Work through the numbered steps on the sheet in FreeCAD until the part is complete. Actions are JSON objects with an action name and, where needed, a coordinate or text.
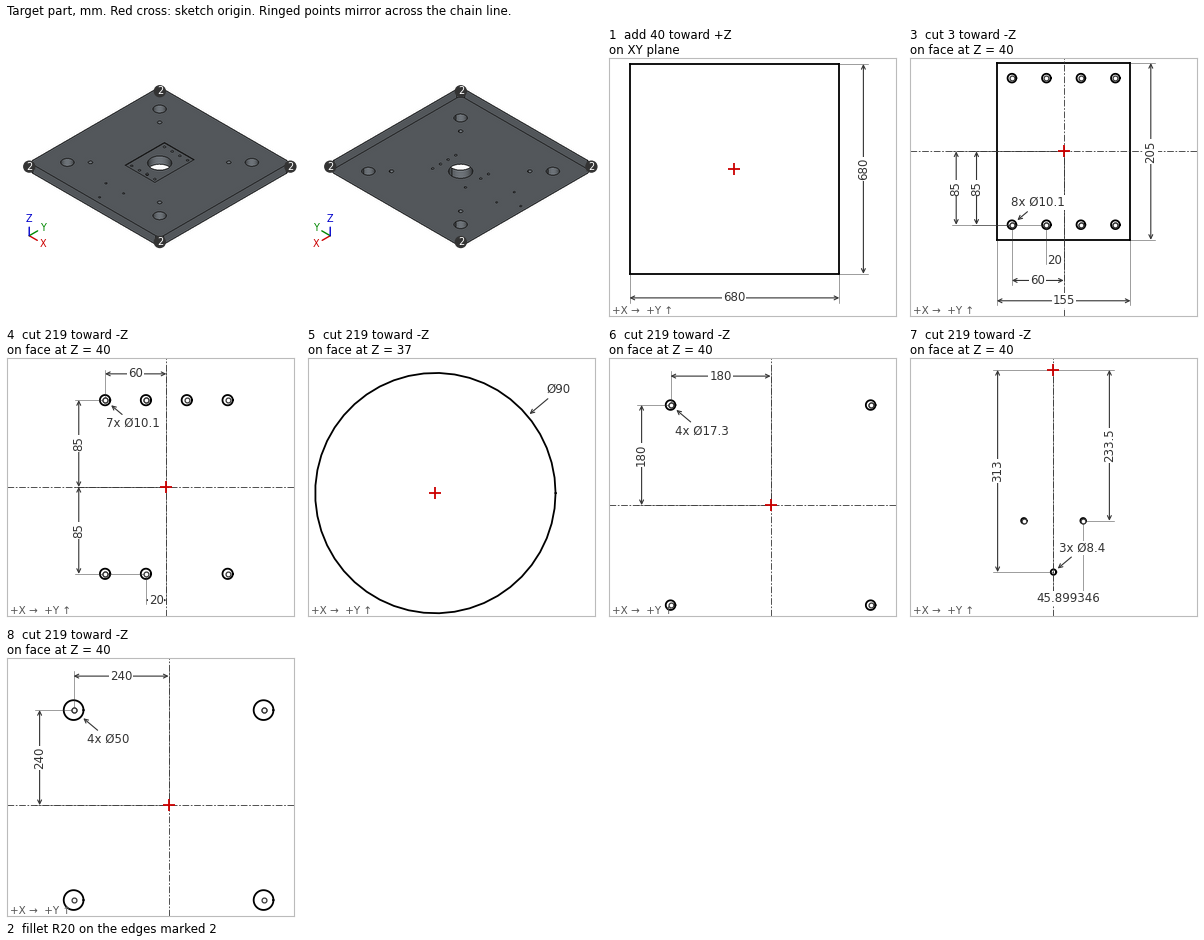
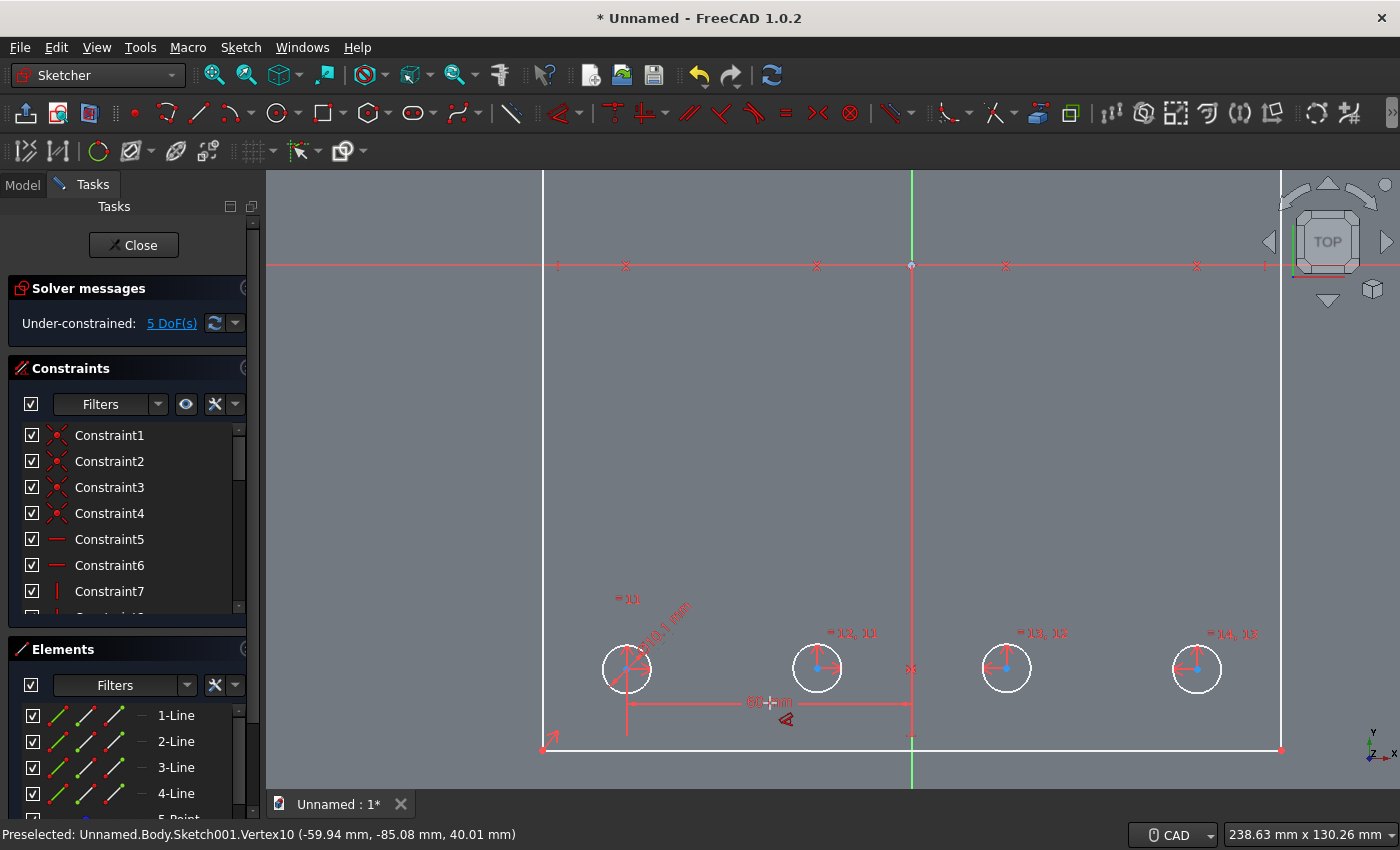
{"action": "left_click", "coordinate": [627, 669]}
{"action": "left_click", "coordinate": [593, 467]}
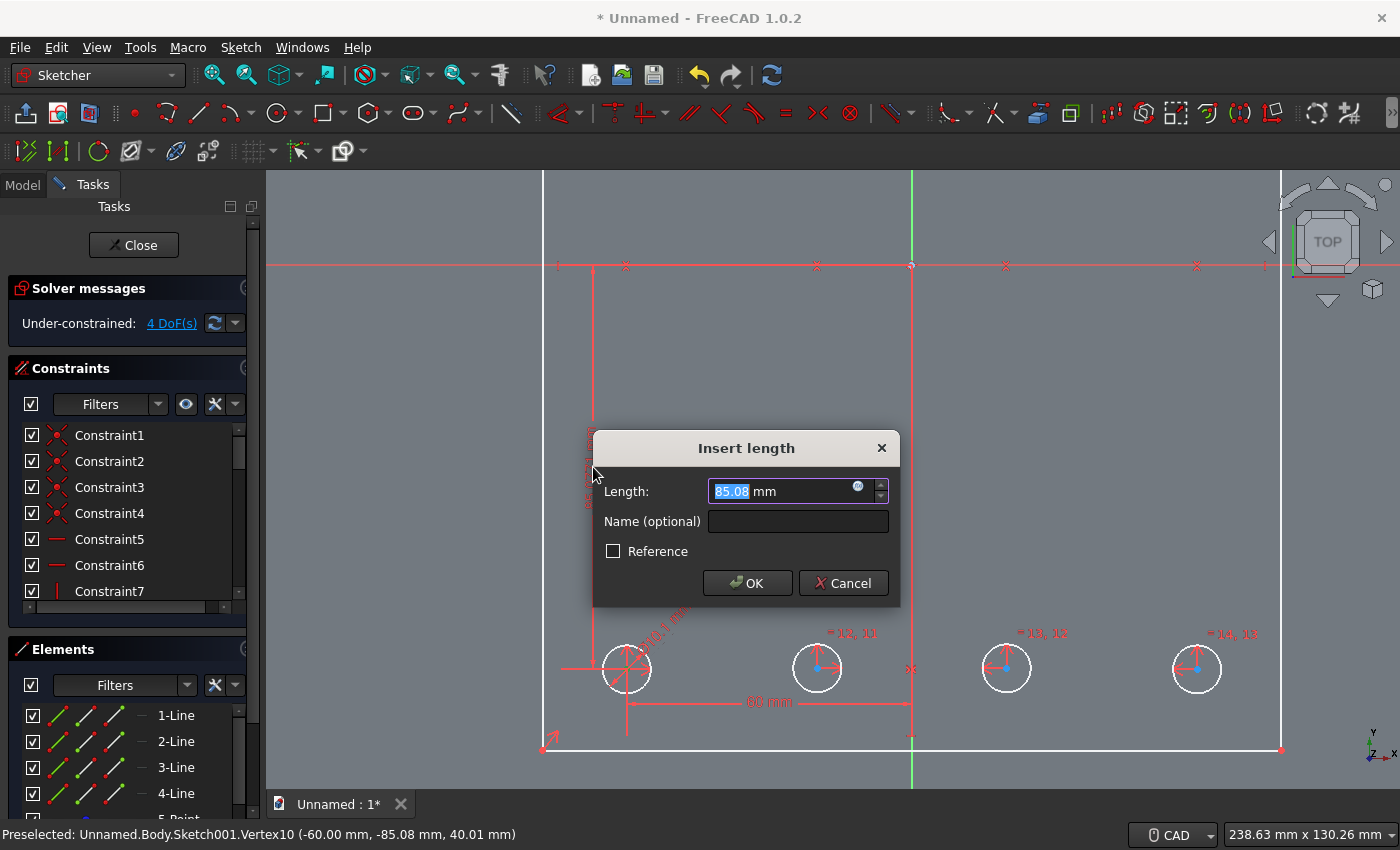
{"action": "type", "text": "85"}
{"action": "key", "text": "Return"}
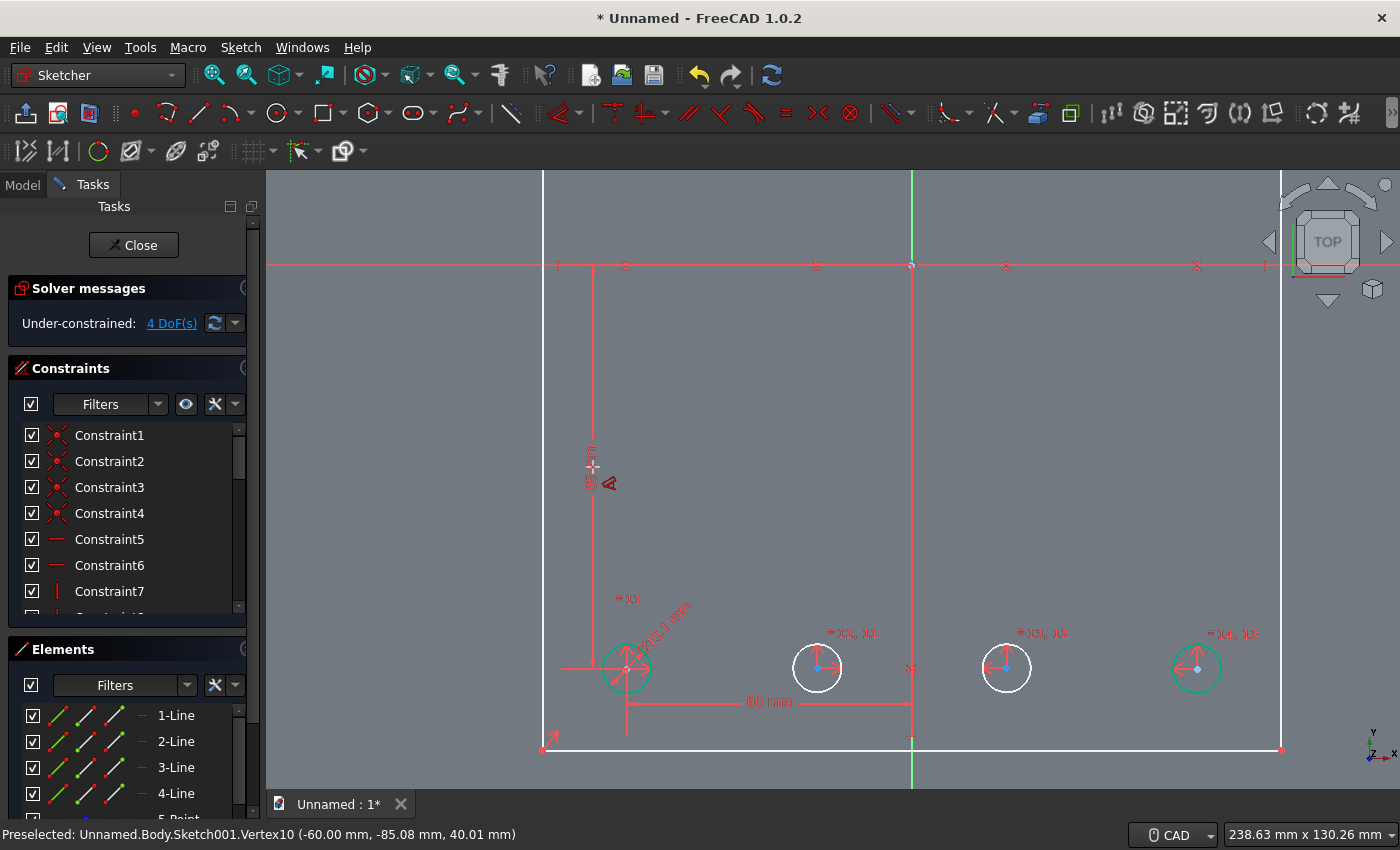
{"action": "left_click", "coordinate": [817, 668]}
{"action": "left_click", "coordinate": [865, 702]}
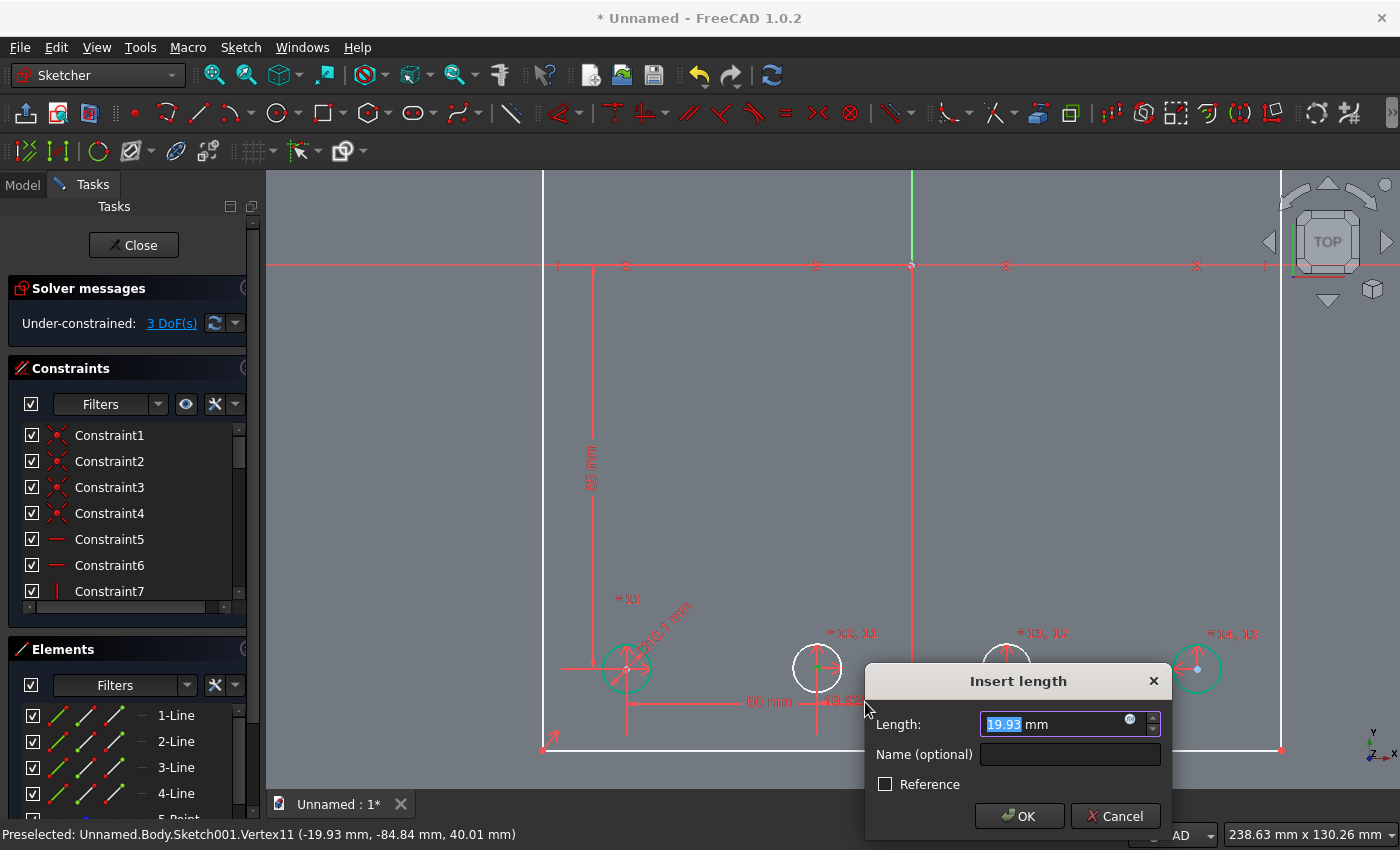
{"action": "type", "text": "20"}
{"action": "key", "text": "Return"}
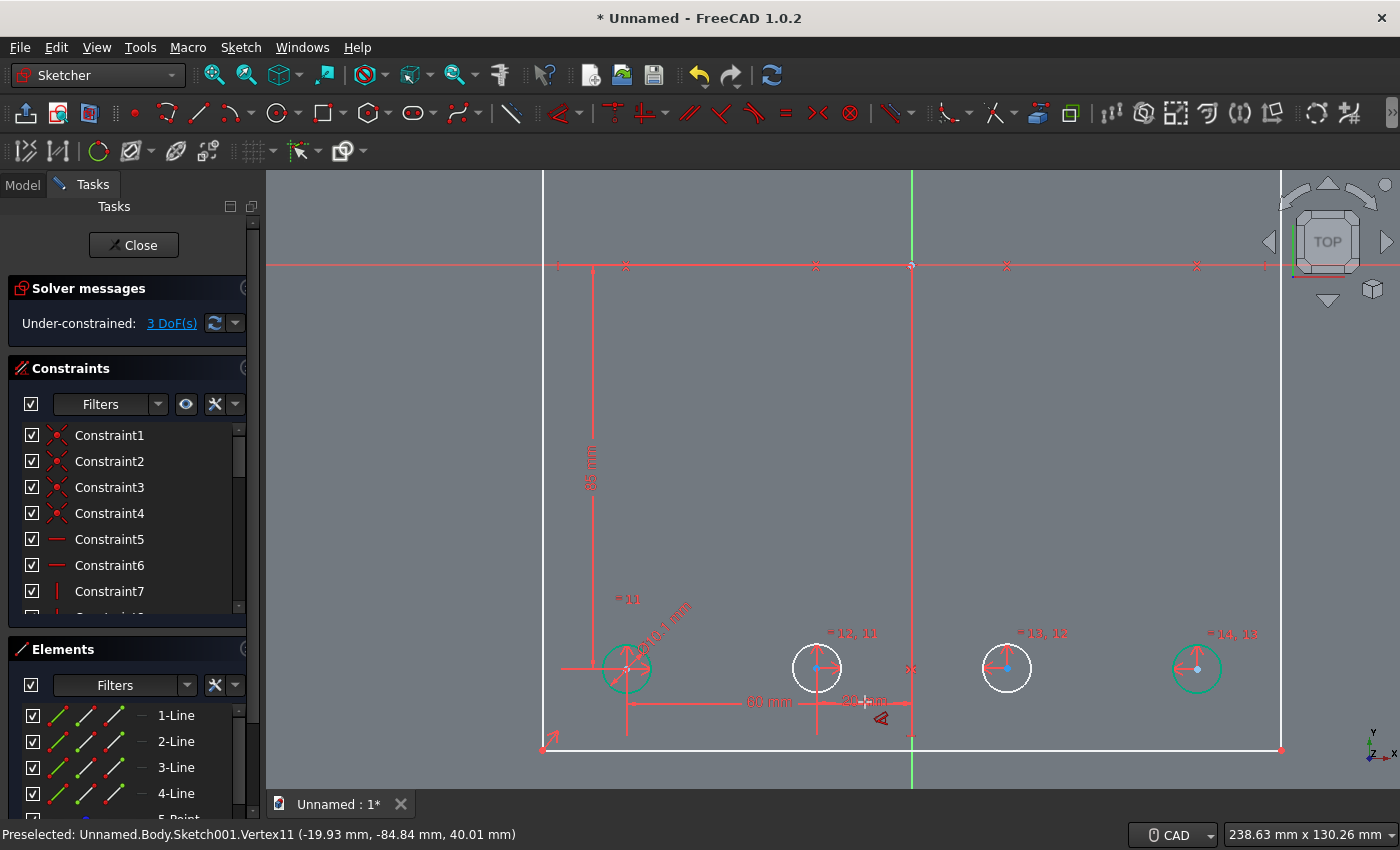
{"action": "left_click", "coordinate": [817, 668]}
{"action": "left_click", "coordinate": [783, 467]}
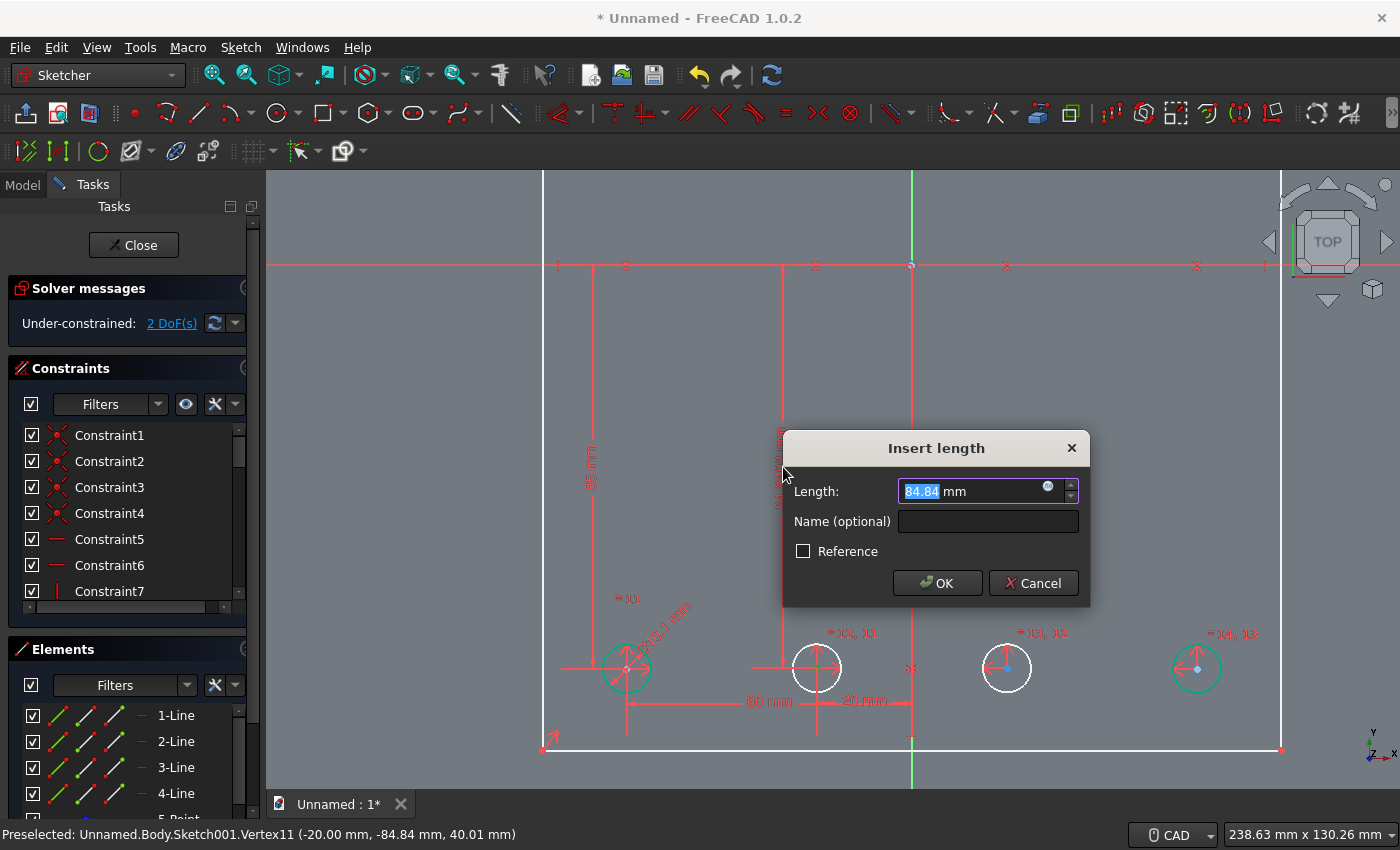
{"action": "type", "text": "85"}
{"action": "key", "text": "Return"}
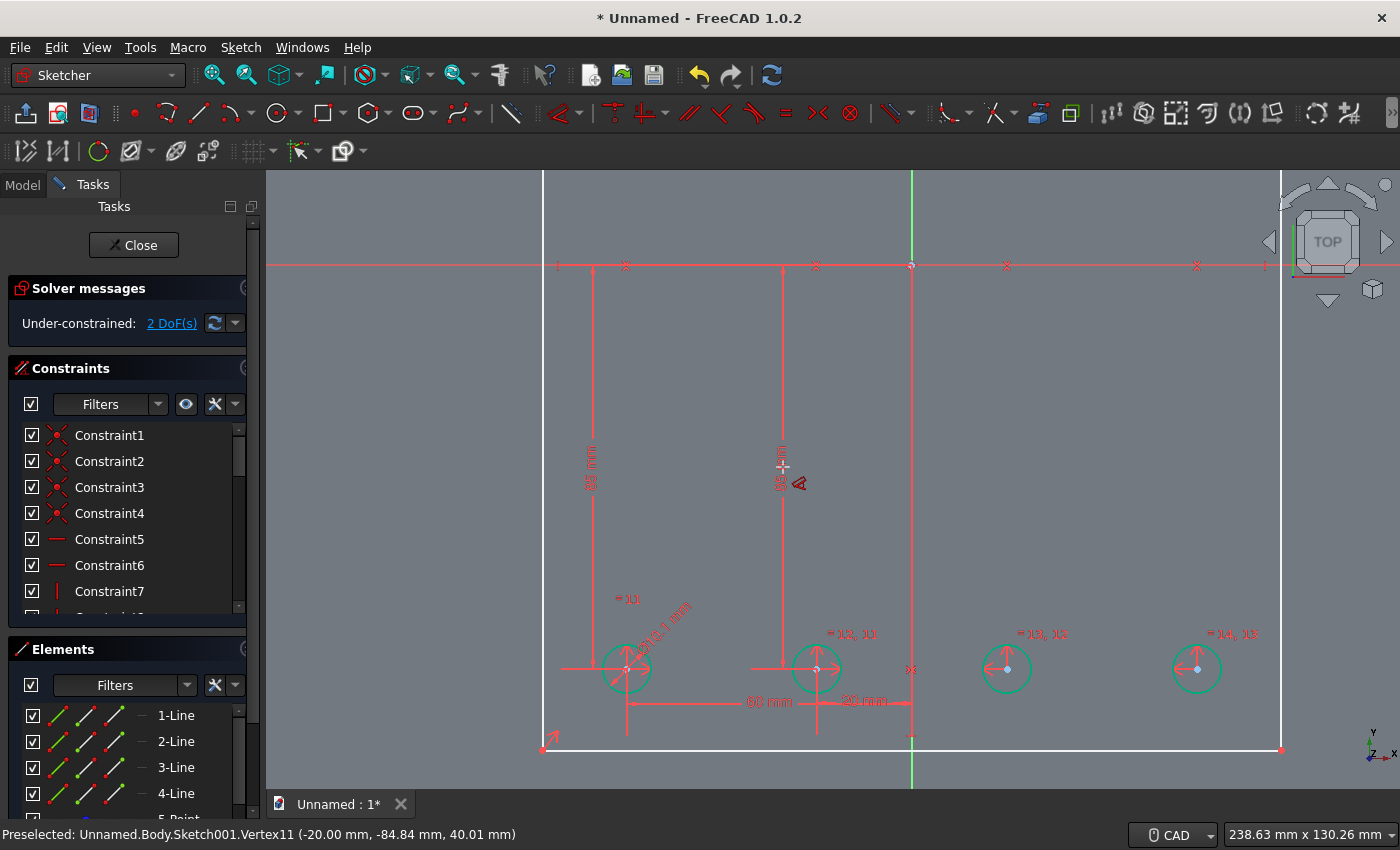
{"action": "left_click", "coordinate": [764, 751]}
{"action": "left_click", "coordinate": [1048, 717]}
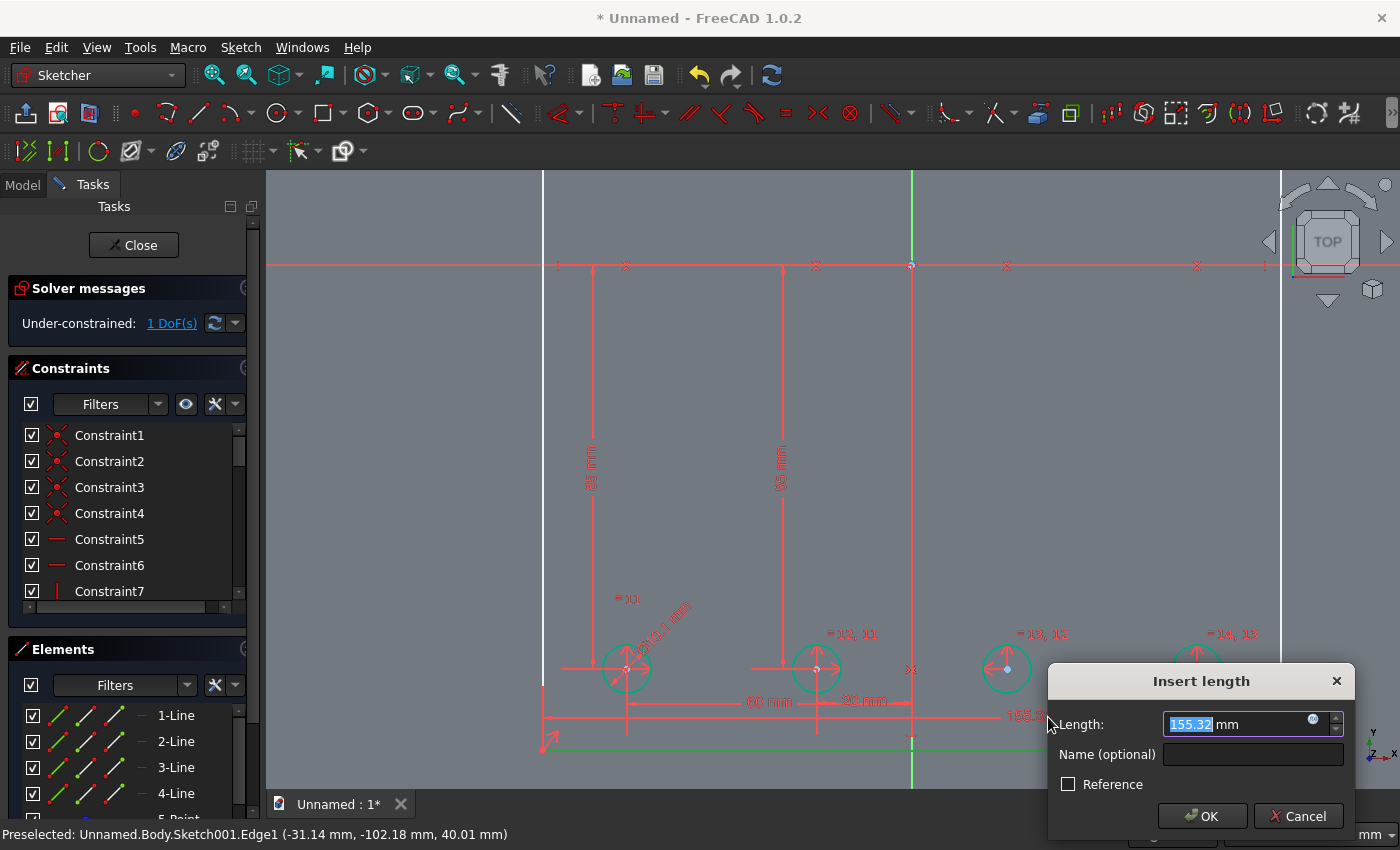
{"action": "type", "text": "155"}
{"action": "key", "text": "Return"}